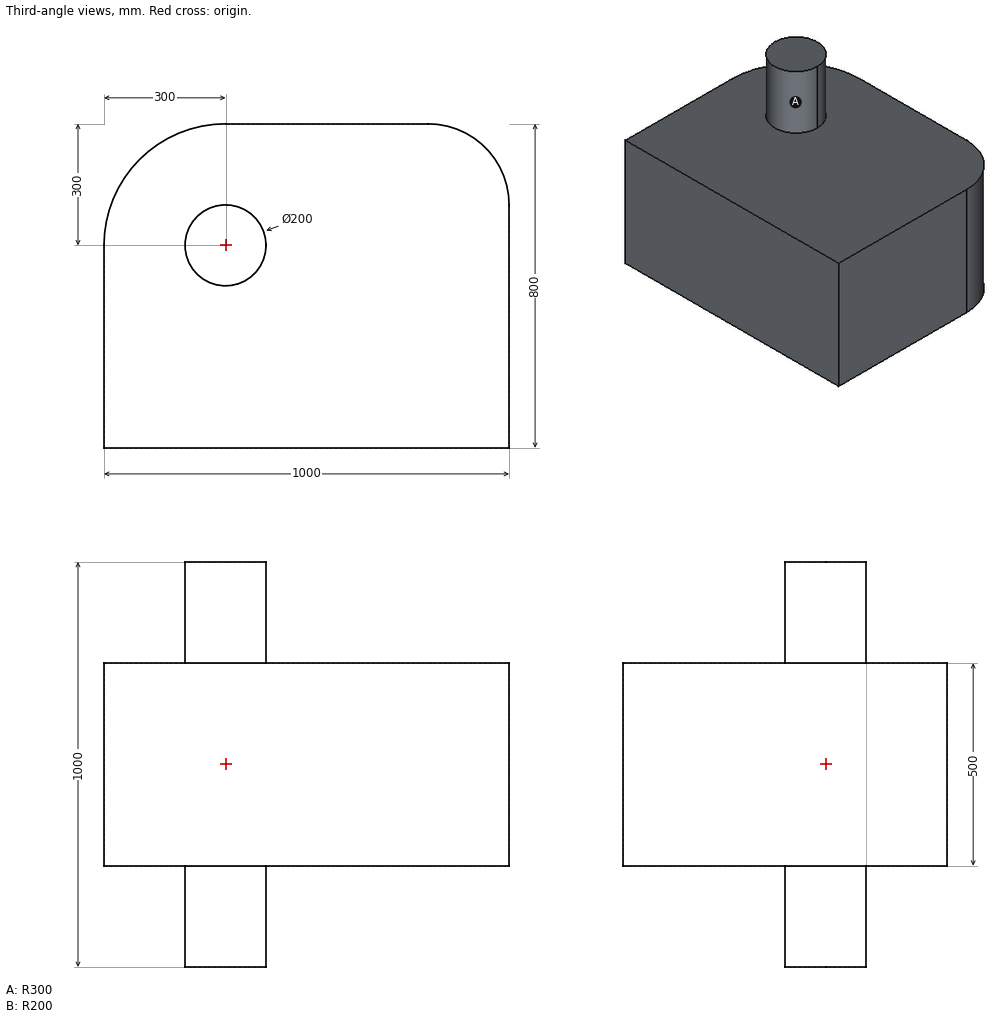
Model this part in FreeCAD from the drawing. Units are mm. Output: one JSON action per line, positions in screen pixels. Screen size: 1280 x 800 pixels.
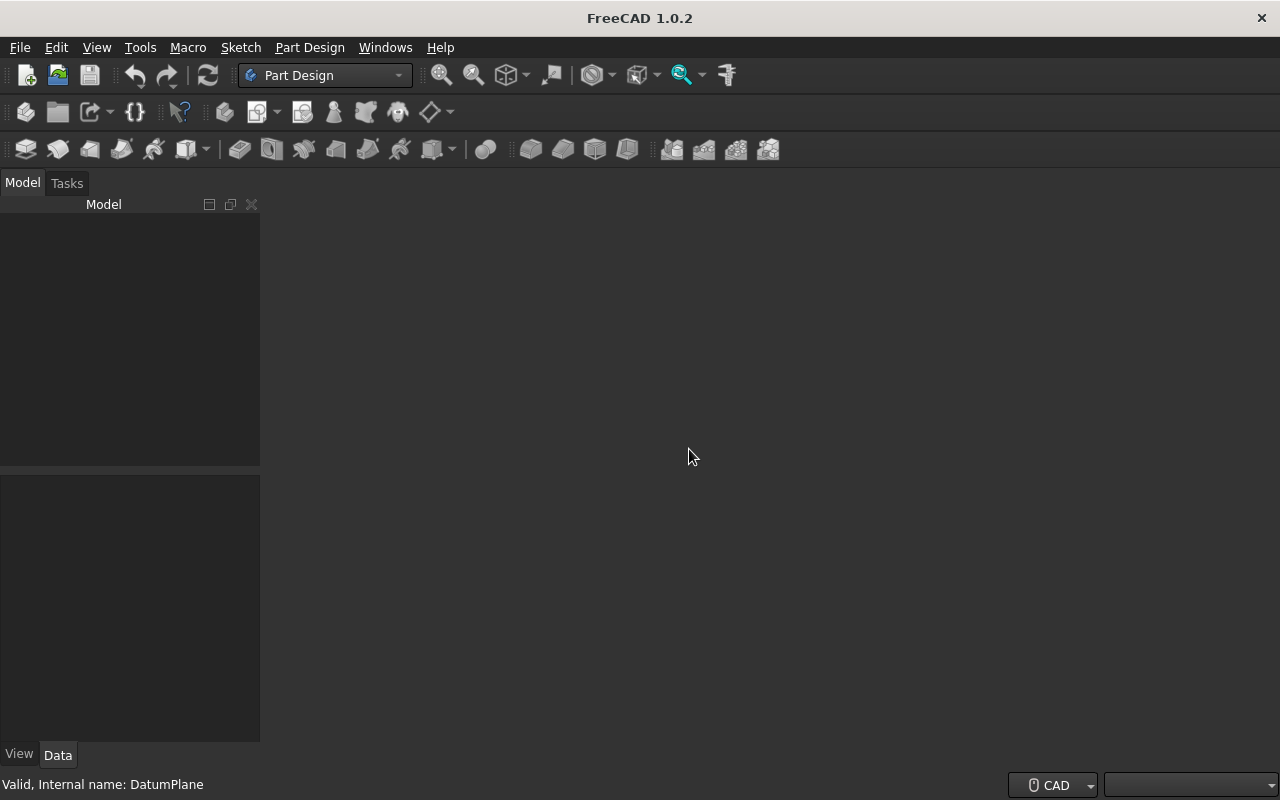
{"action": "left_click", "coordinate": [26, 76]}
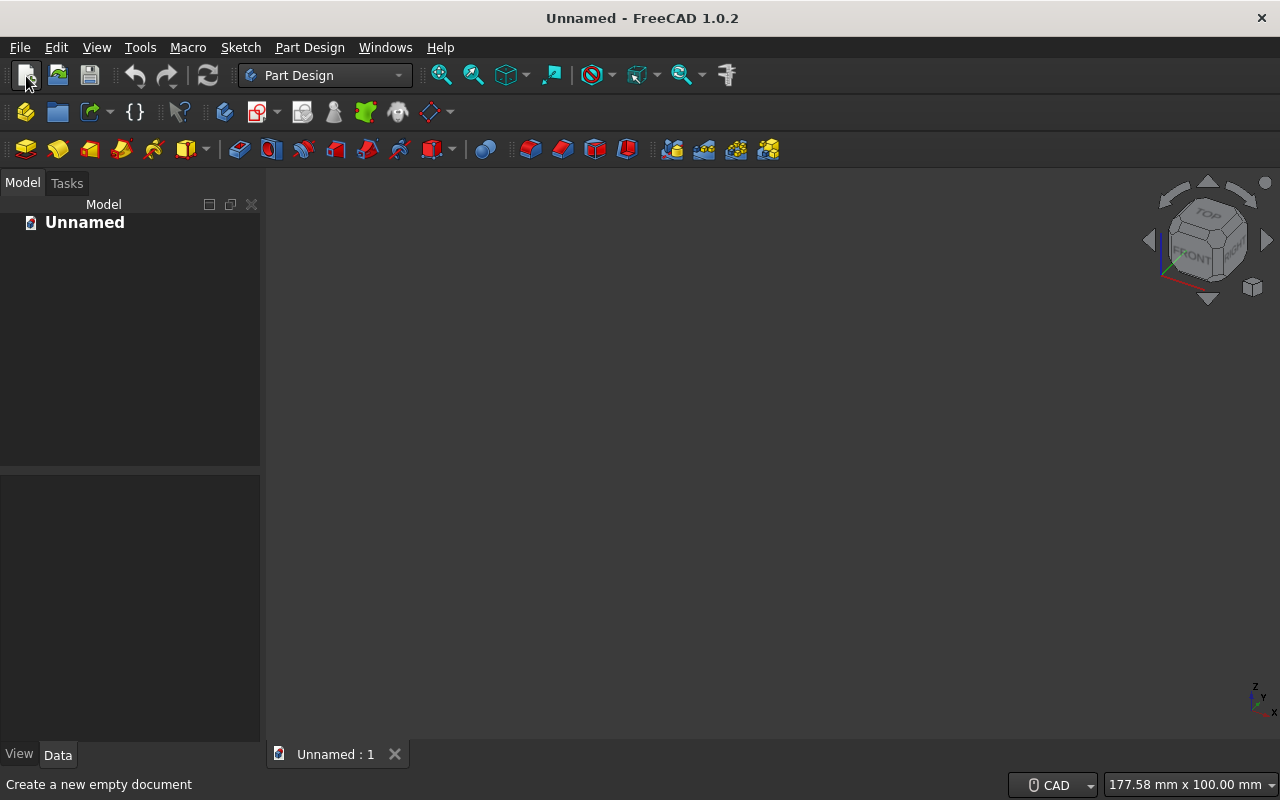
{"action": "left_click", "coordinate": [258, 112]}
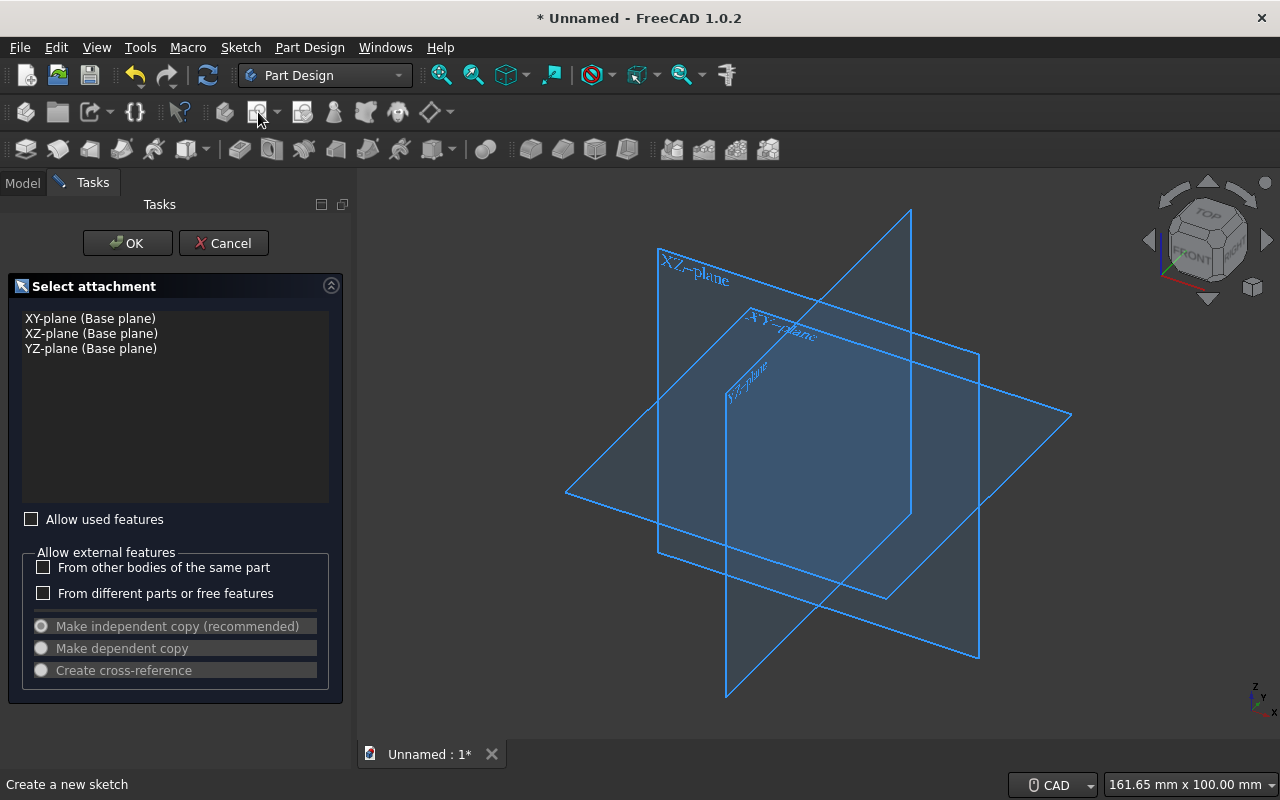
{"action": "left_click", "coordinate": [82, 318]}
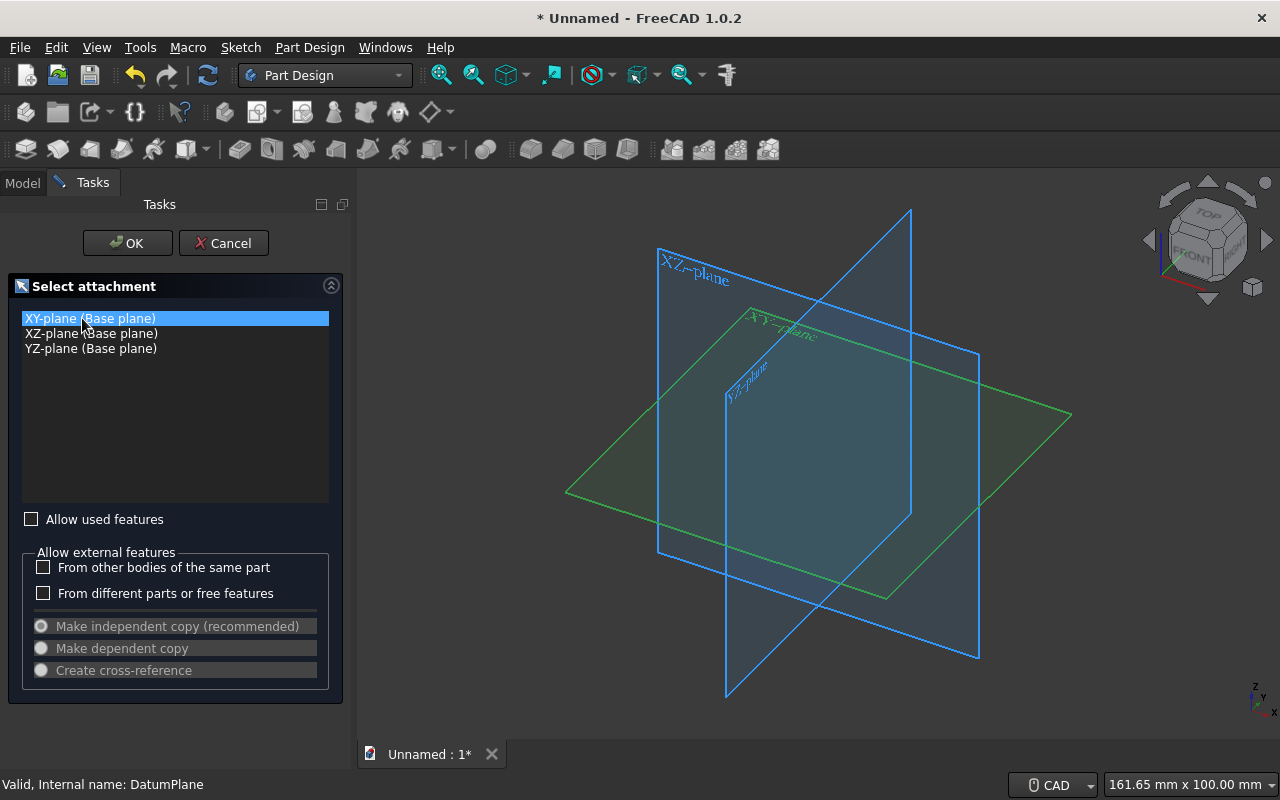
{"action": "left_click", "coordinate": [128, 243]}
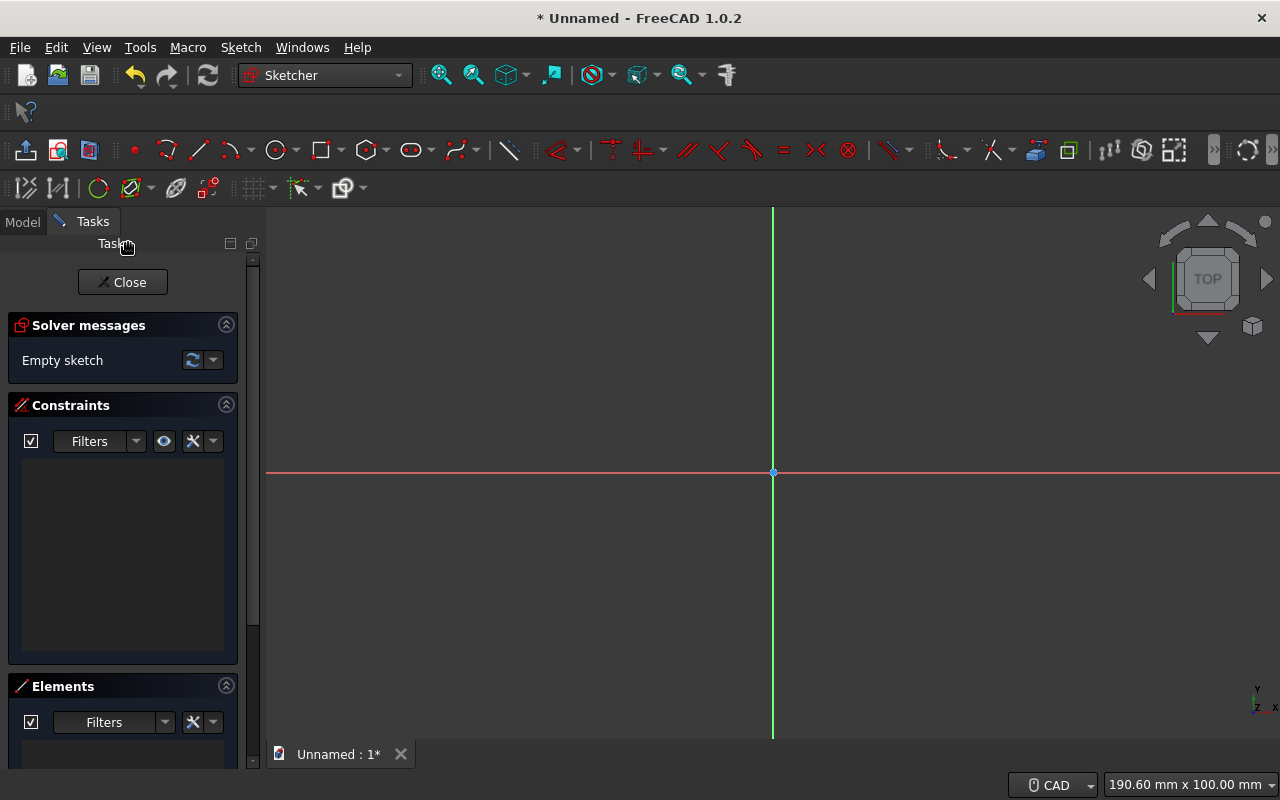
{"action": "scroll", "coordinate": [614, 430], "scroll_direction": "down", "scroll_amount": 13}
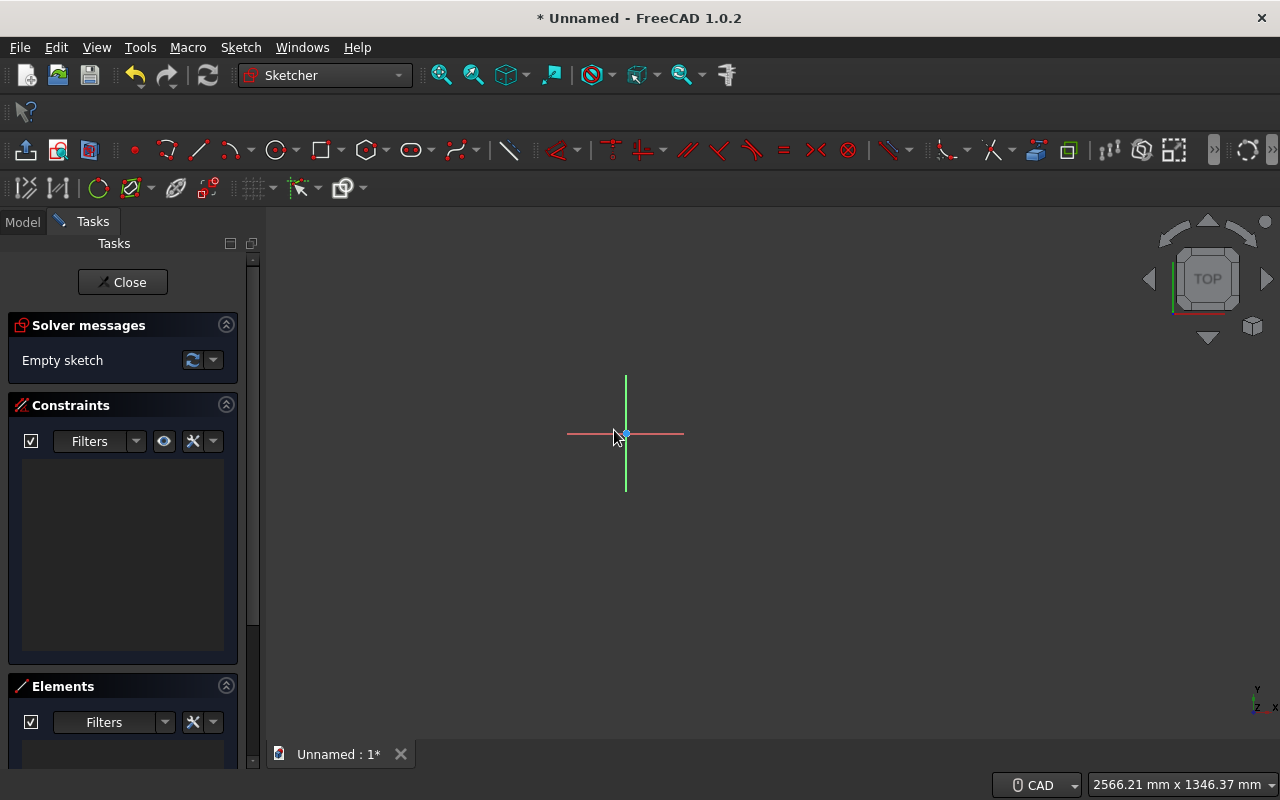
{"action": "left_click", "coordinate": [322, 150]}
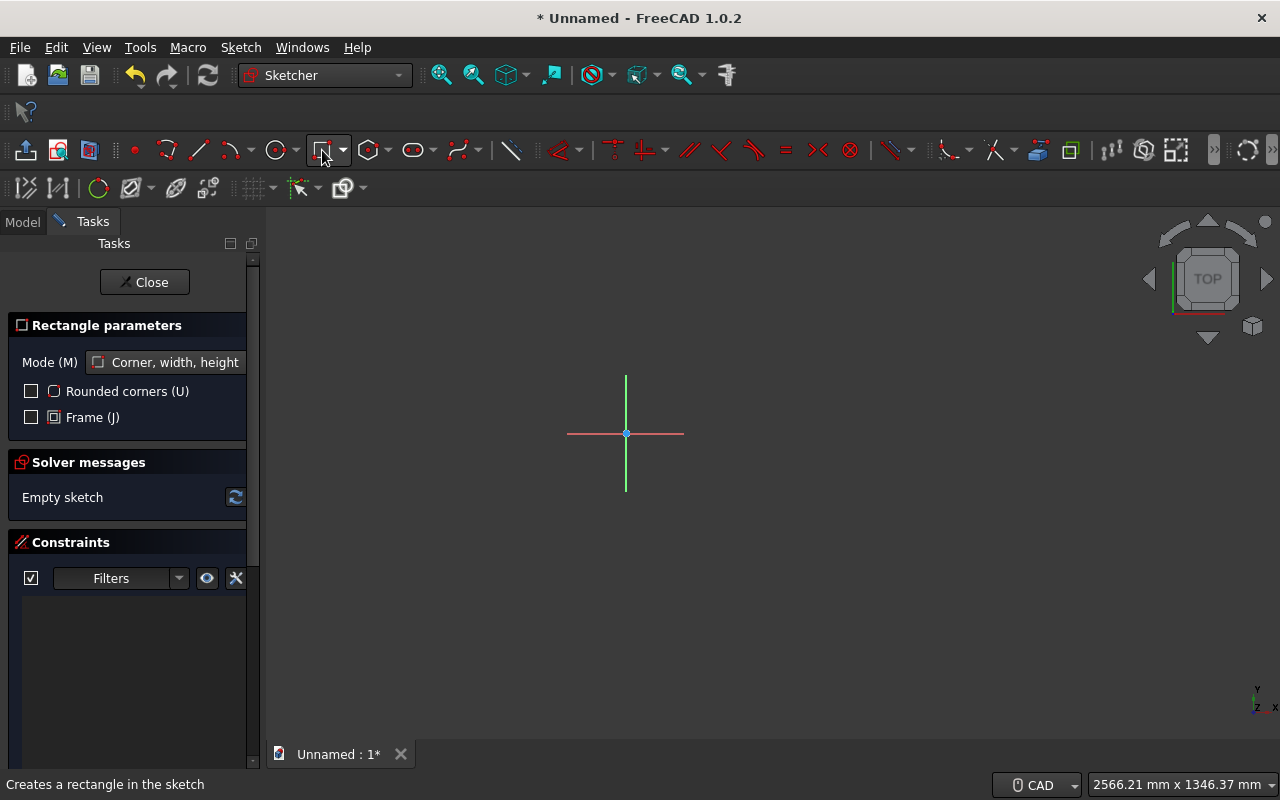
{"action": "left_click", "coordinate": [508, 315]}
{"action": "mouse_move", "coordinate": [903, 631]}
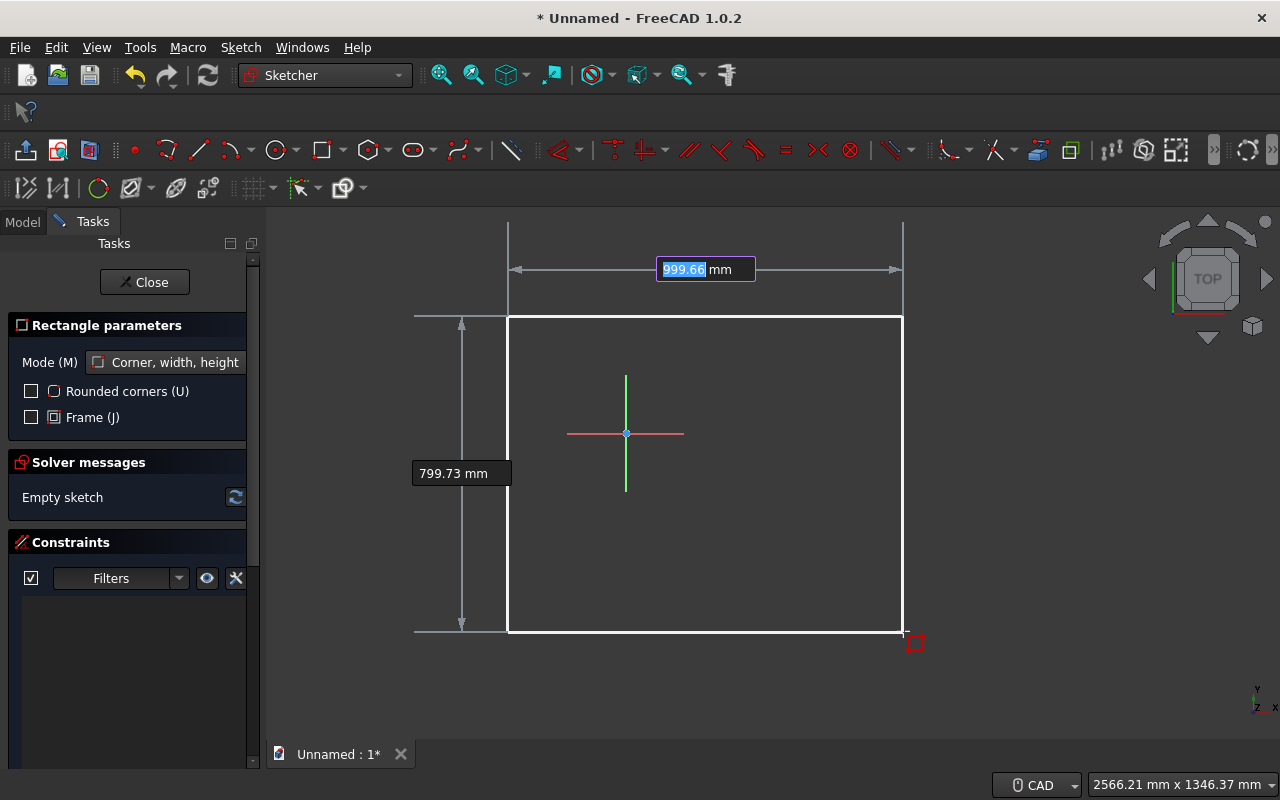
{"action": "type", "text": "1000"}
{"action": "key", "text": "Tab"}
{"action": "type", "text": "800"}
{"action": "key", "text": "Return"}
{"action": "key", "text": "Escape"}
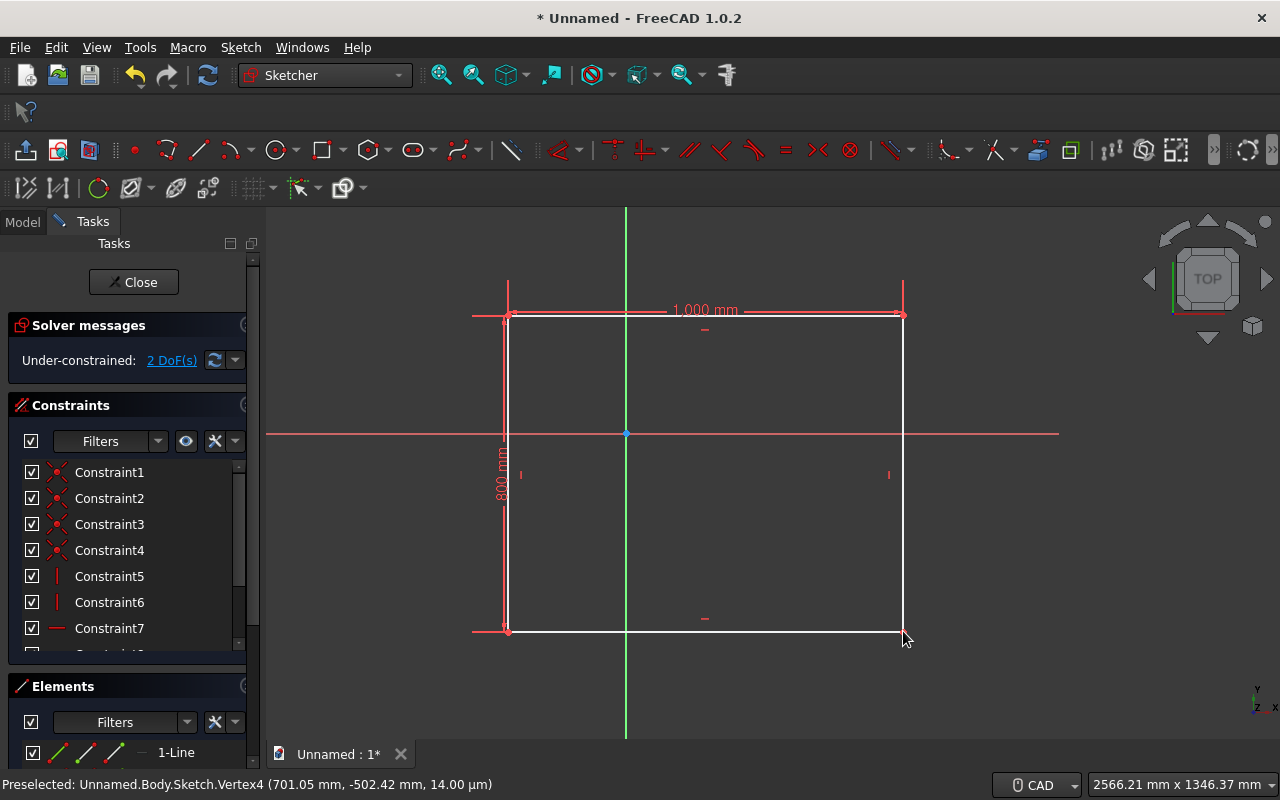
{"action": "left_click", "coordinate": [508, 316]}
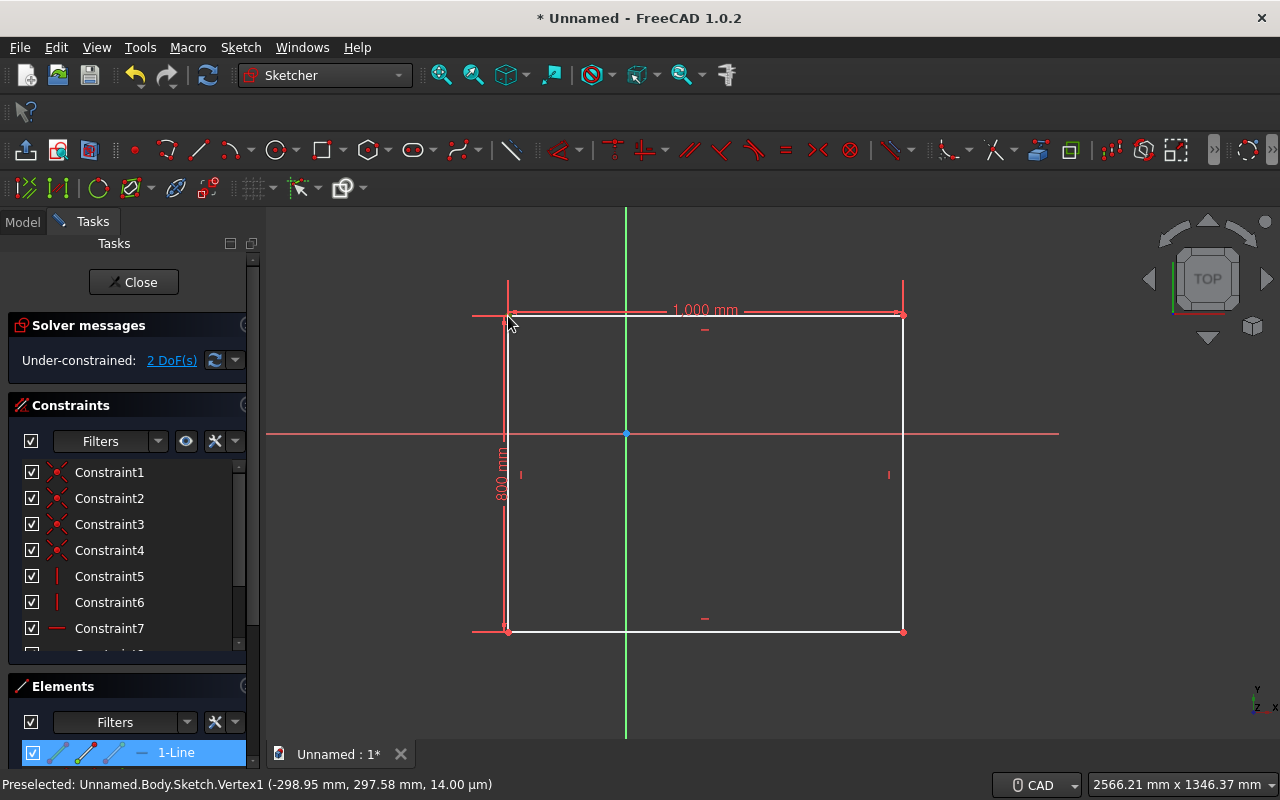
{"action": "left_click", "coordinate": [582, 150]}